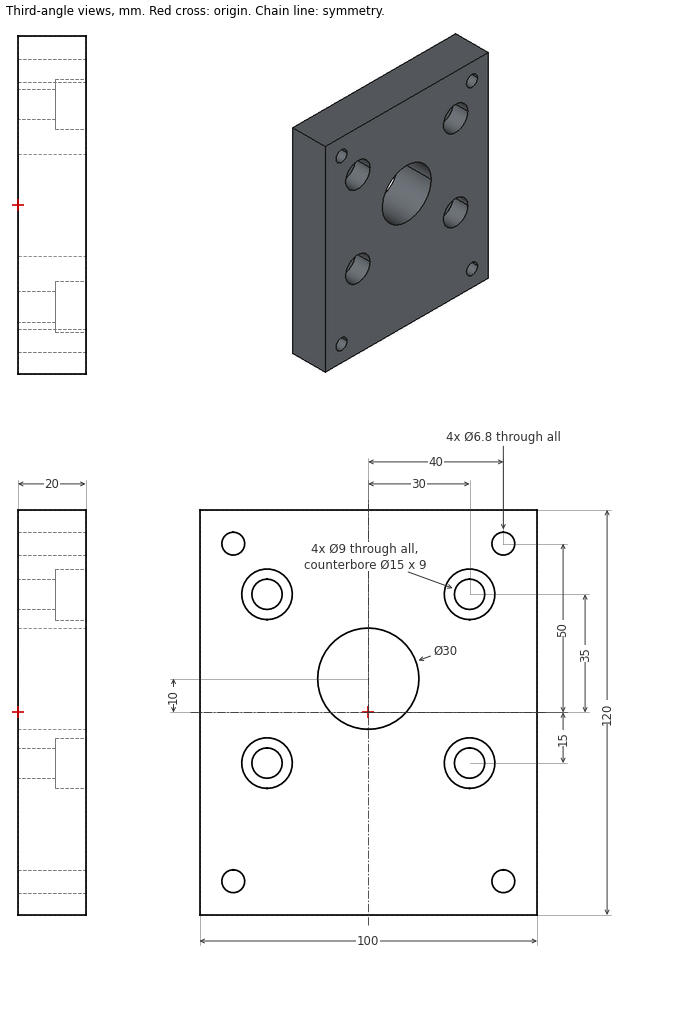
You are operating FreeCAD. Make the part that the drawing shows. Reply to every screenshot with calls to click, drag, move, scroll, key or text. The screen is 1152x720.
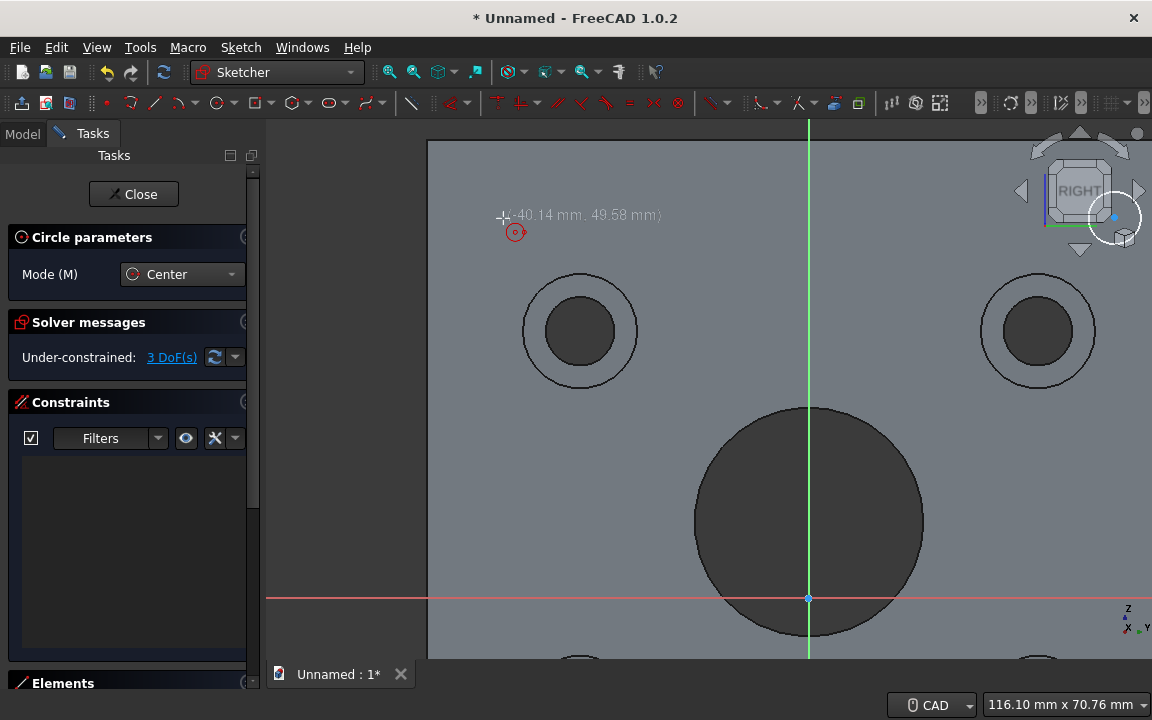
click(504, 217)
click(522, 198)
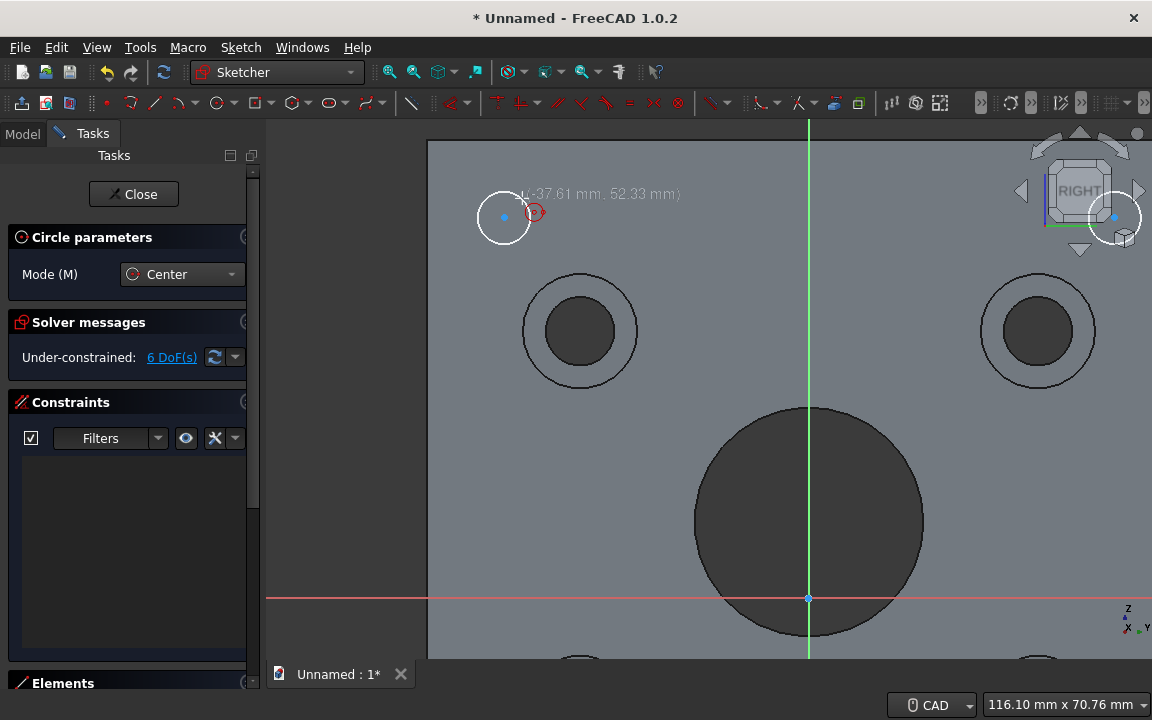
scroll(503, 218, down, 4)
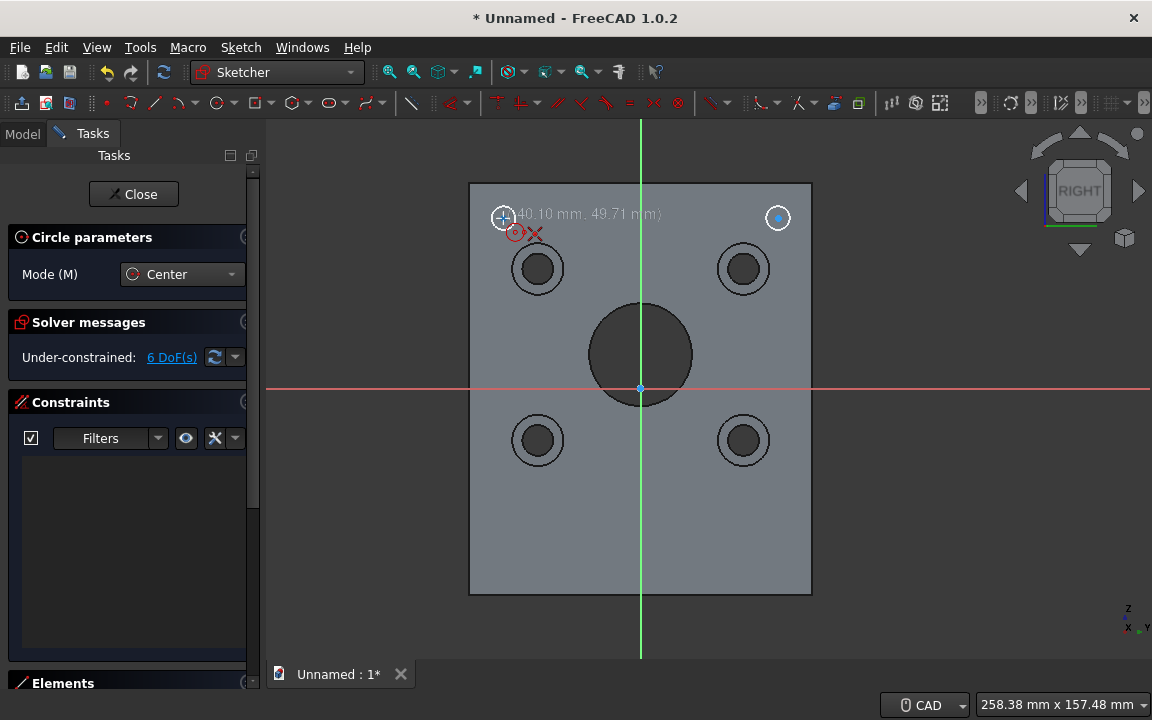
scroll(503, 560, up, 4)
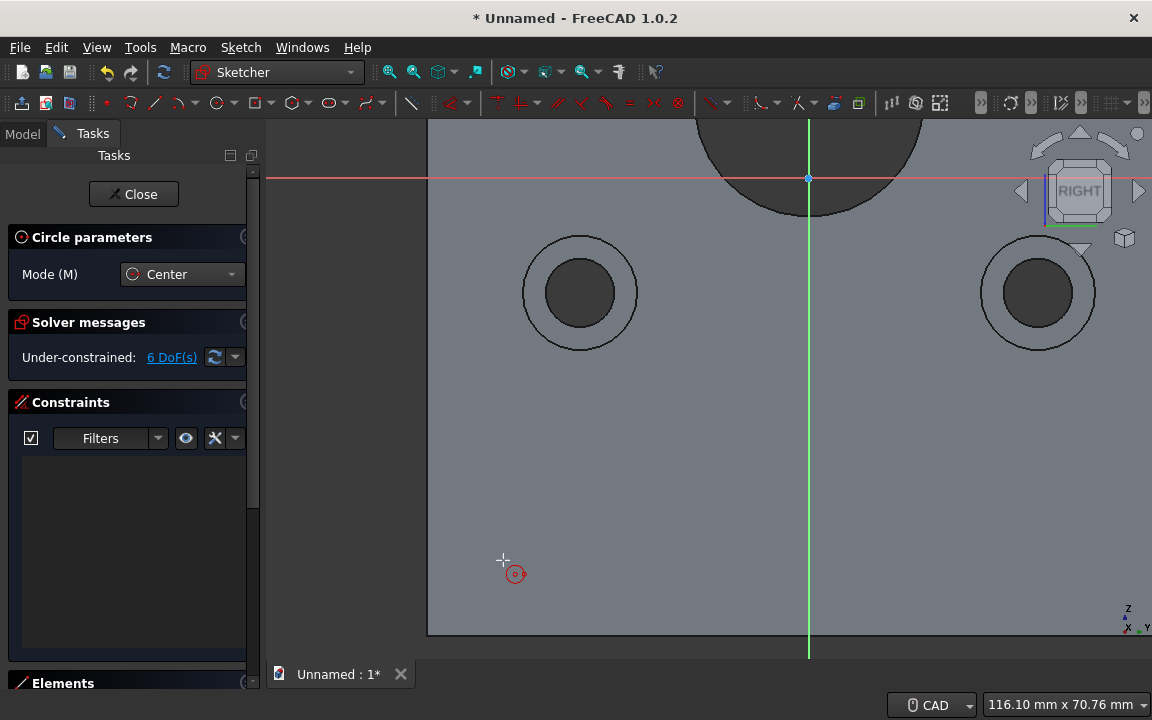
click(504, 560)
click(522, 542)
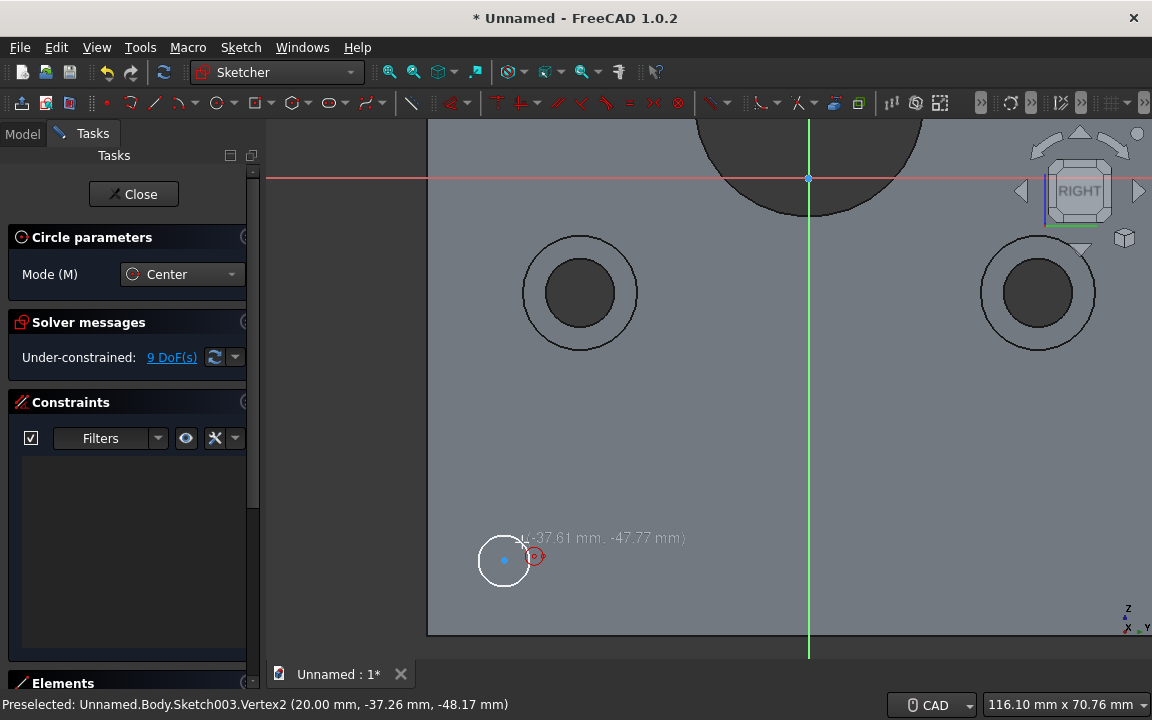
scroll(503, 561, down, 4)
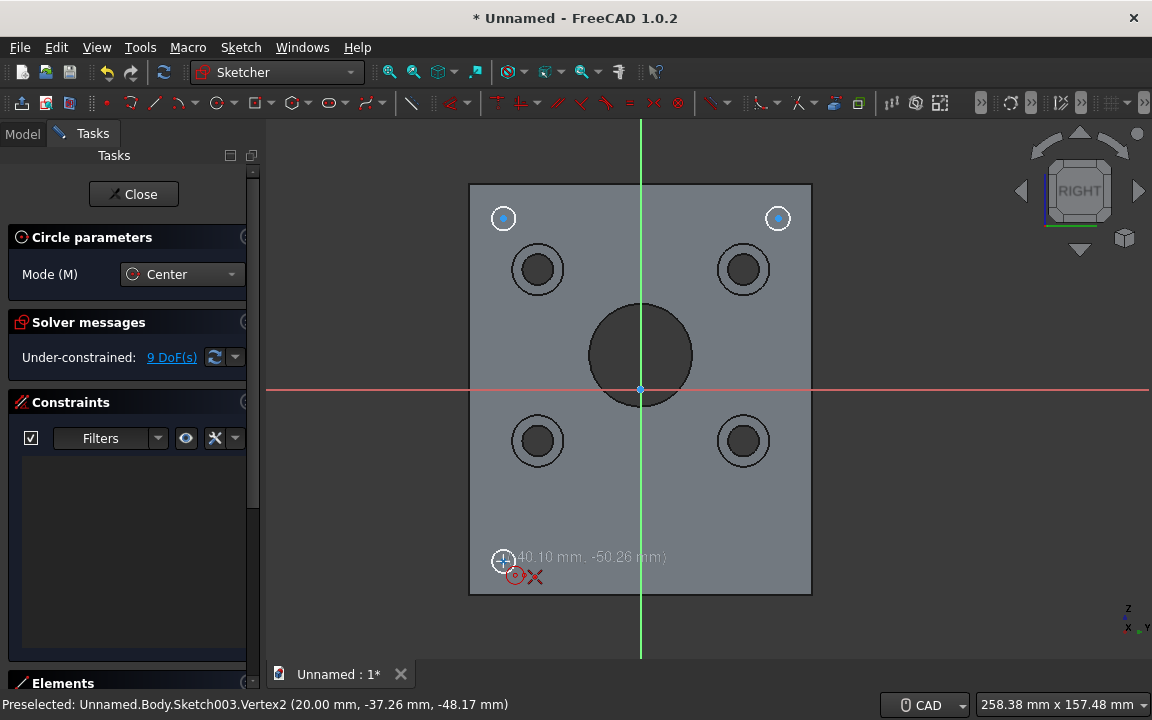
scroll(778, 561, up, 4)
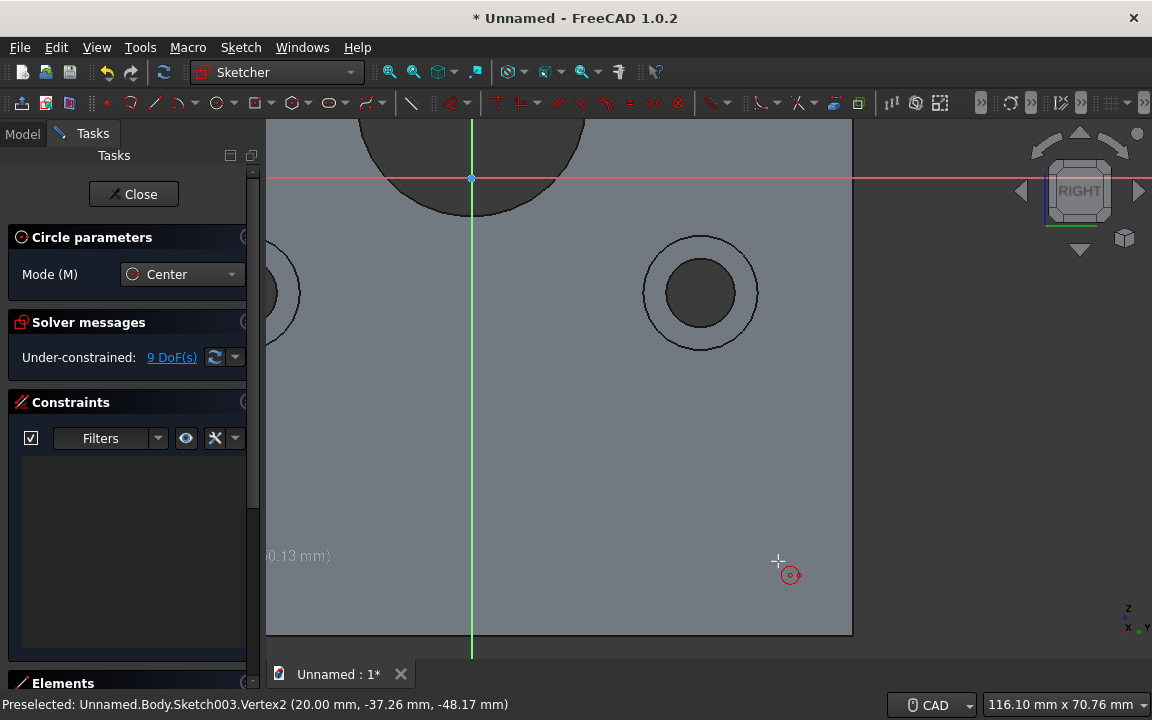
click(777, 560)
click(795, 542)
key(Escape)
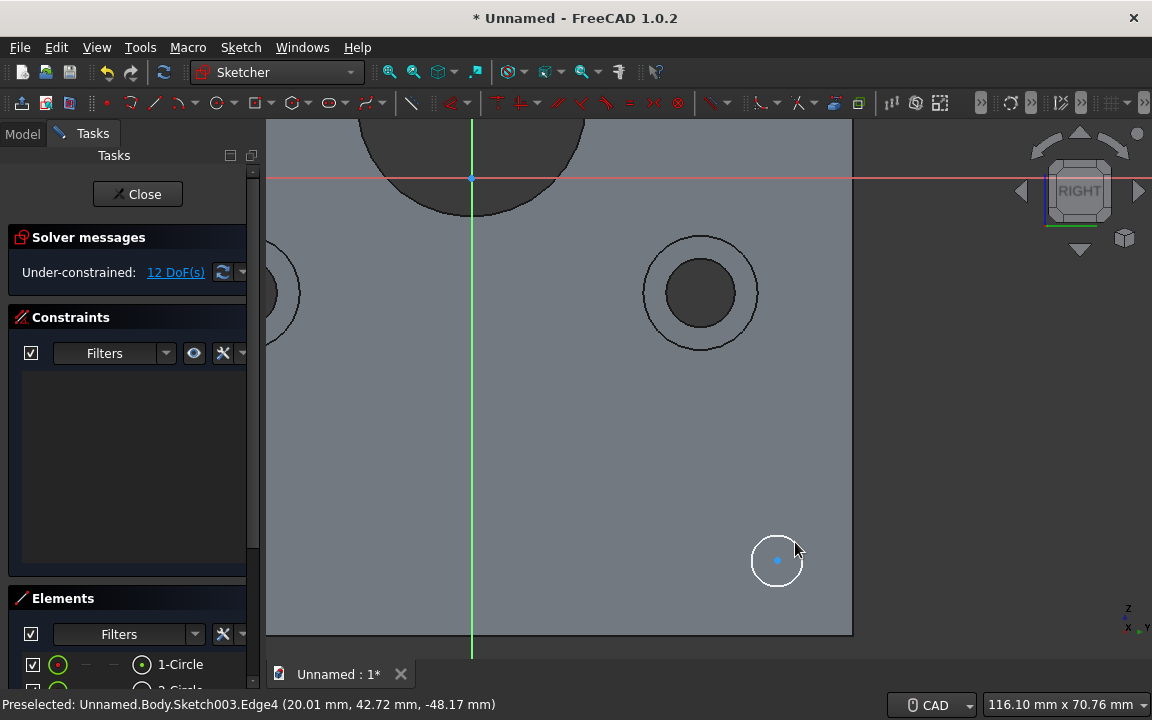
scroll(778, 561, down, 4)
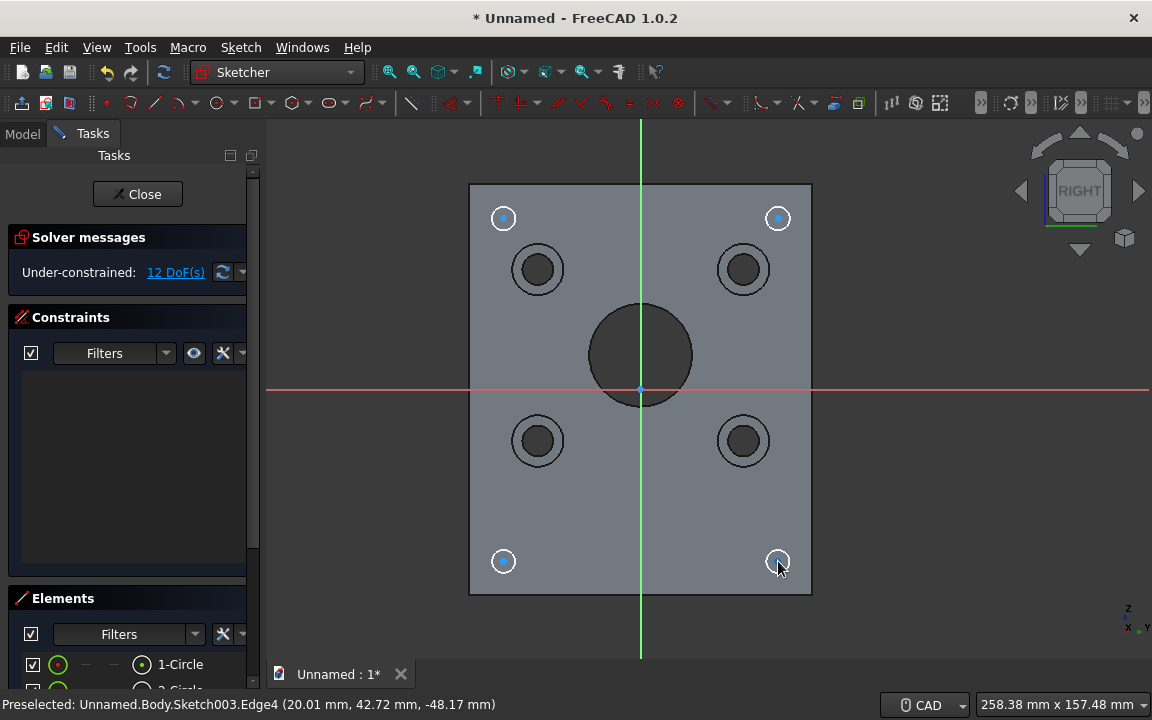
click(786, 210)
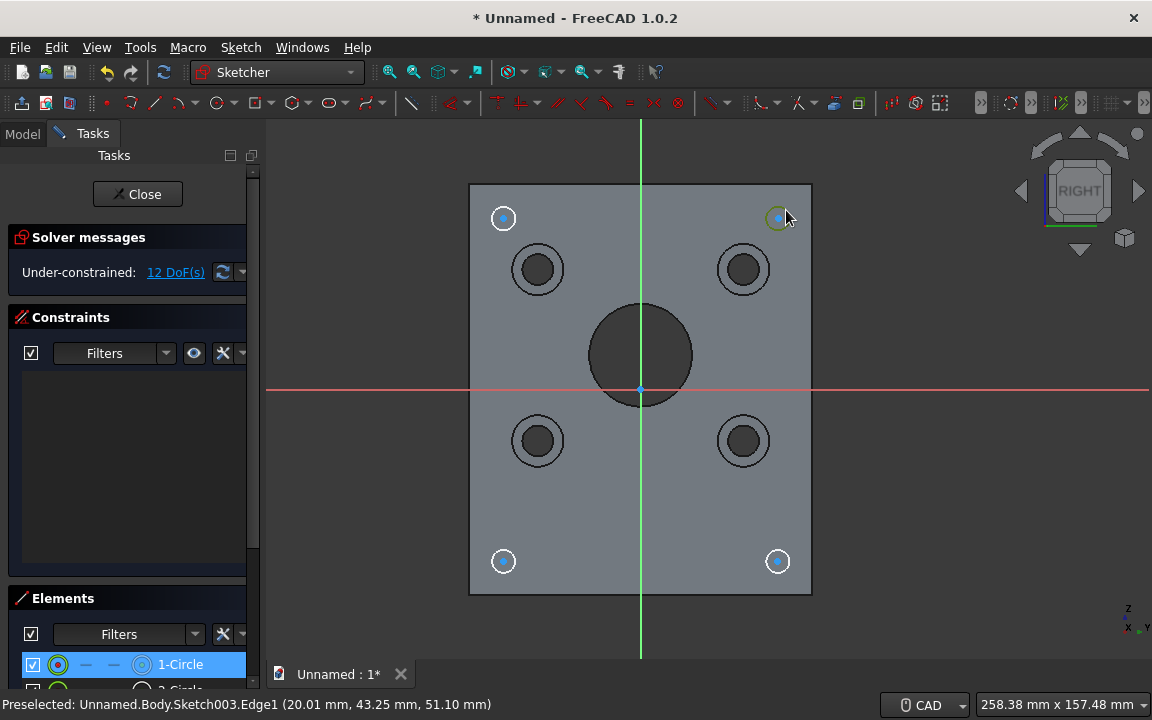
click(512, 210)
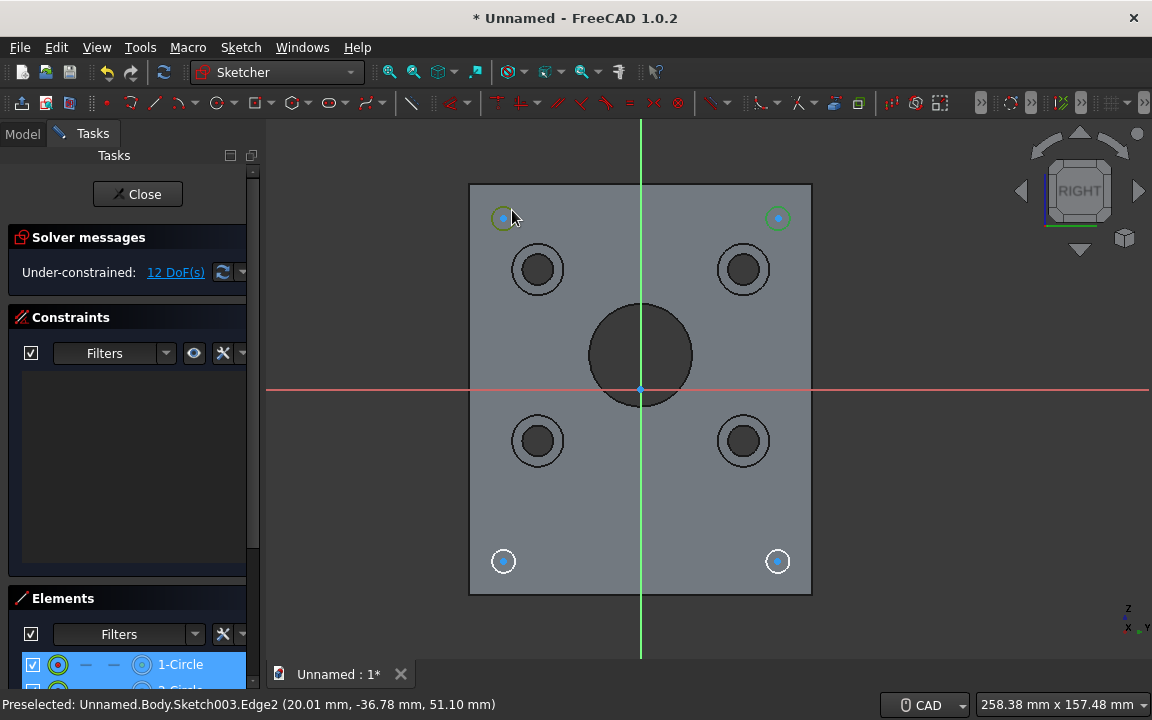
click(512, 553)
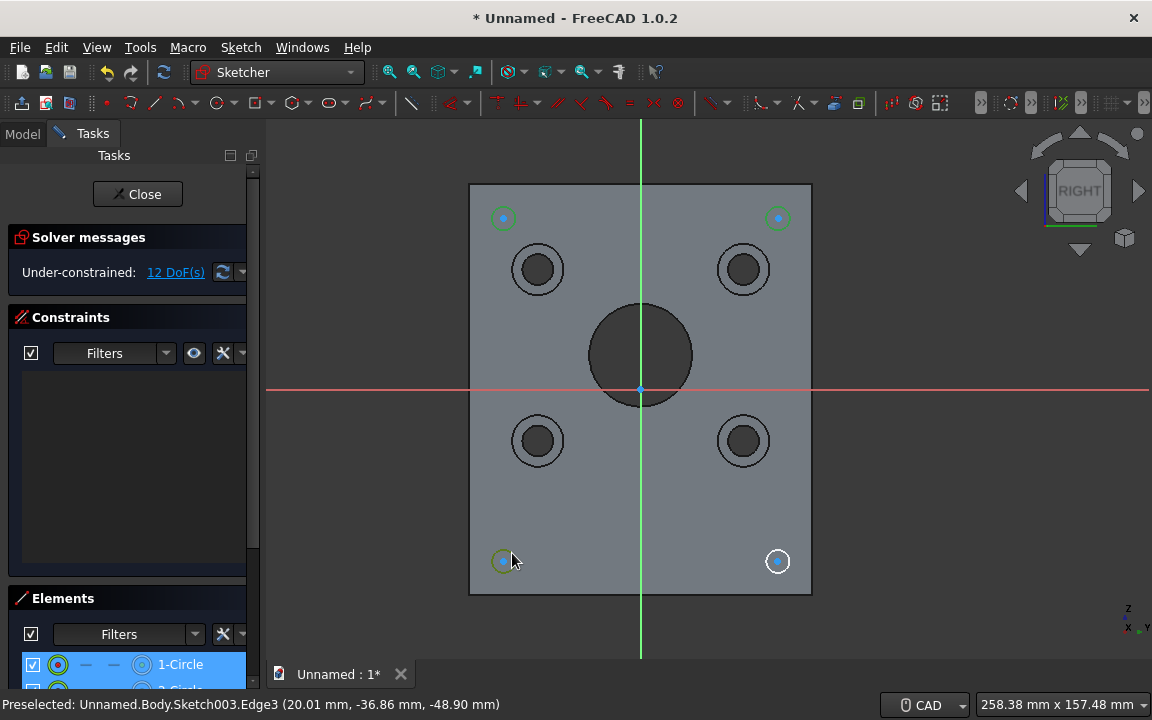
click(786, 553)